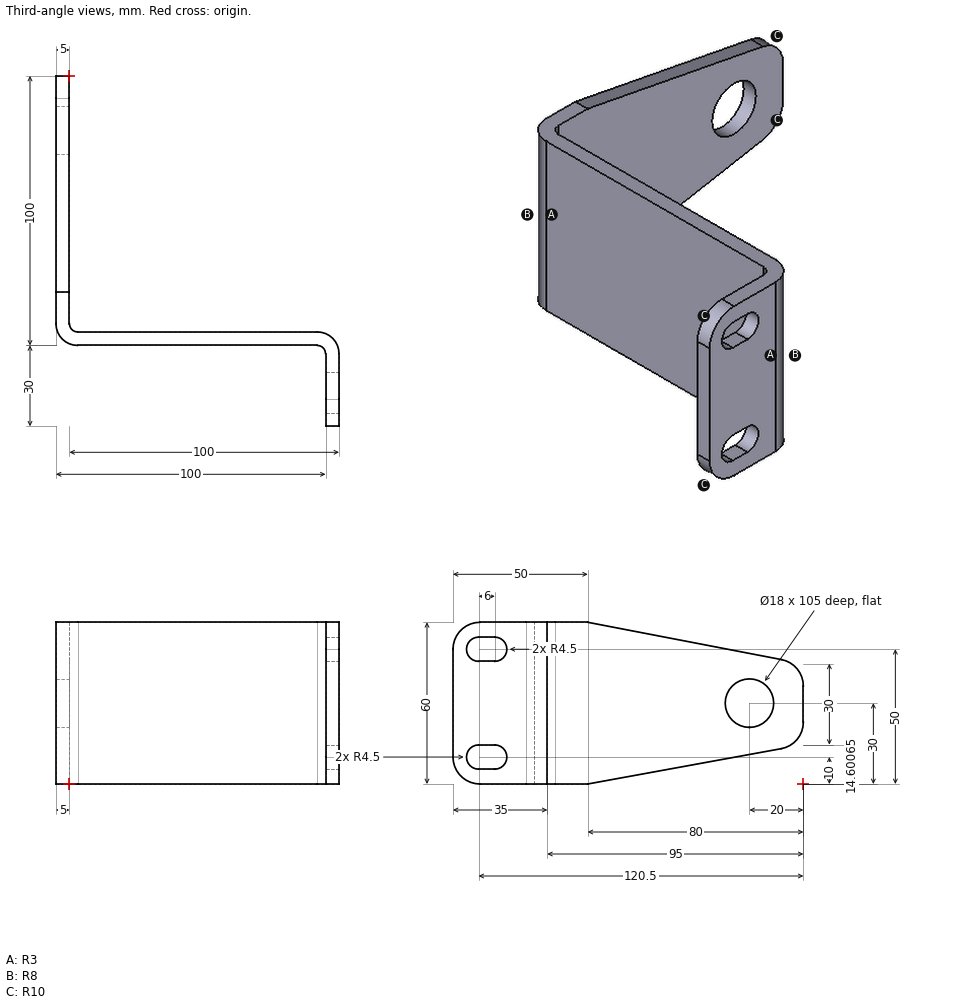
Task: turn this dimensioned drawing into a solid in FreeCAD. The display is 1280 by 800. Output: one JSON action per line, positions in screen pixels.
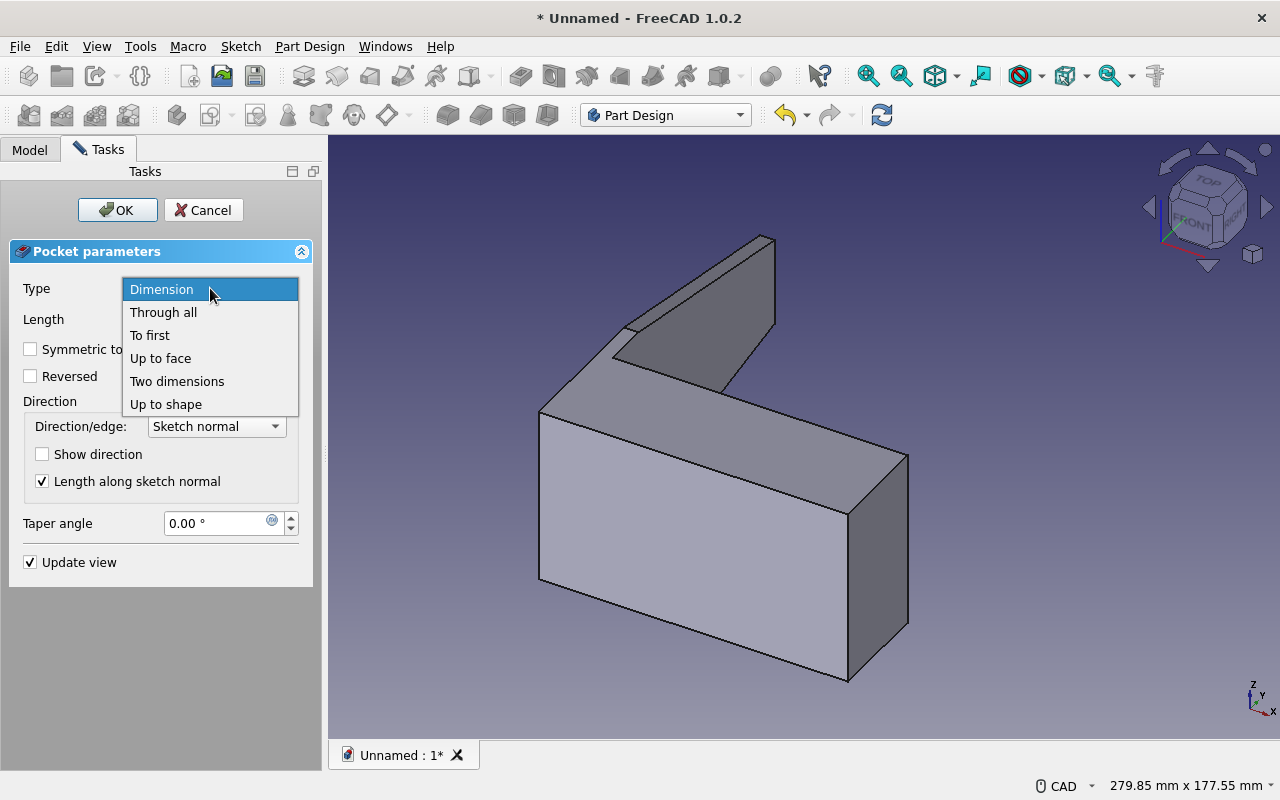
{"action": "left_click", "coordinate": [208, 312]}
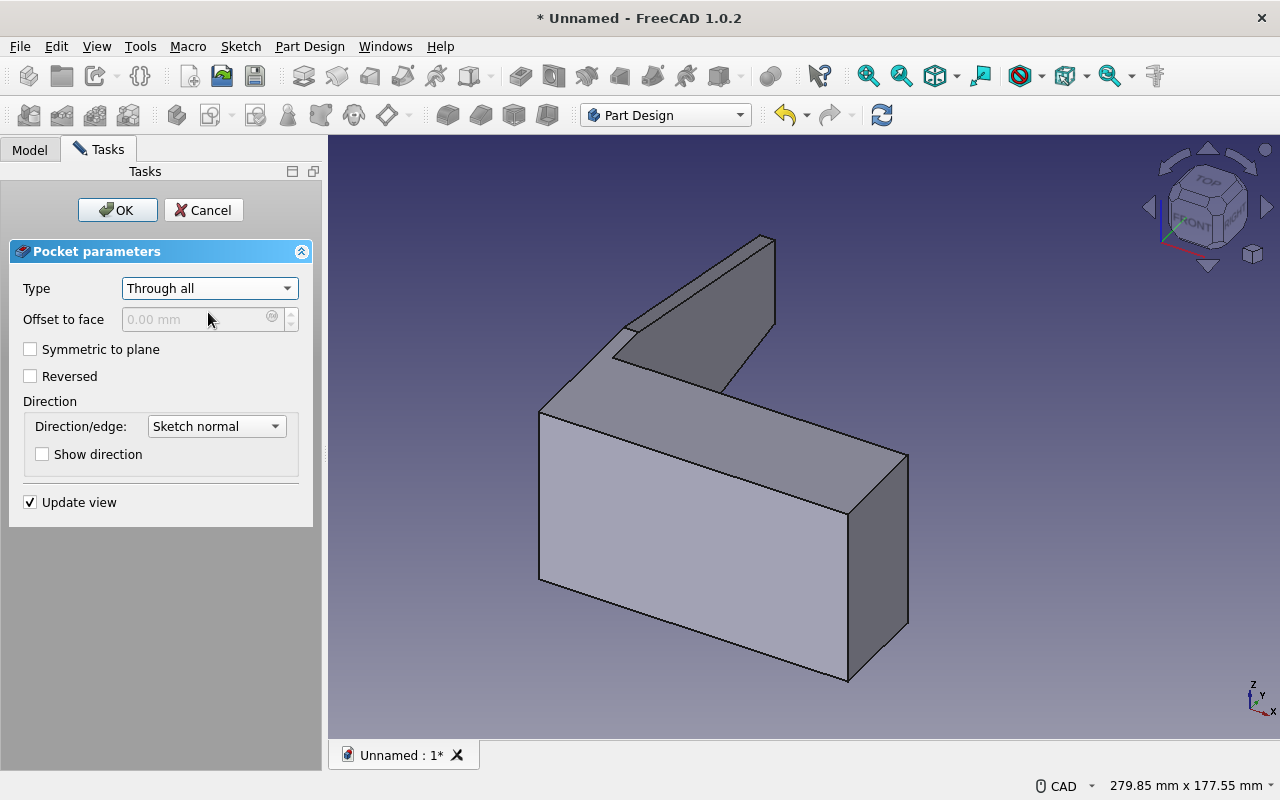
{"action": "left_click", "coordinate": [31, 376]}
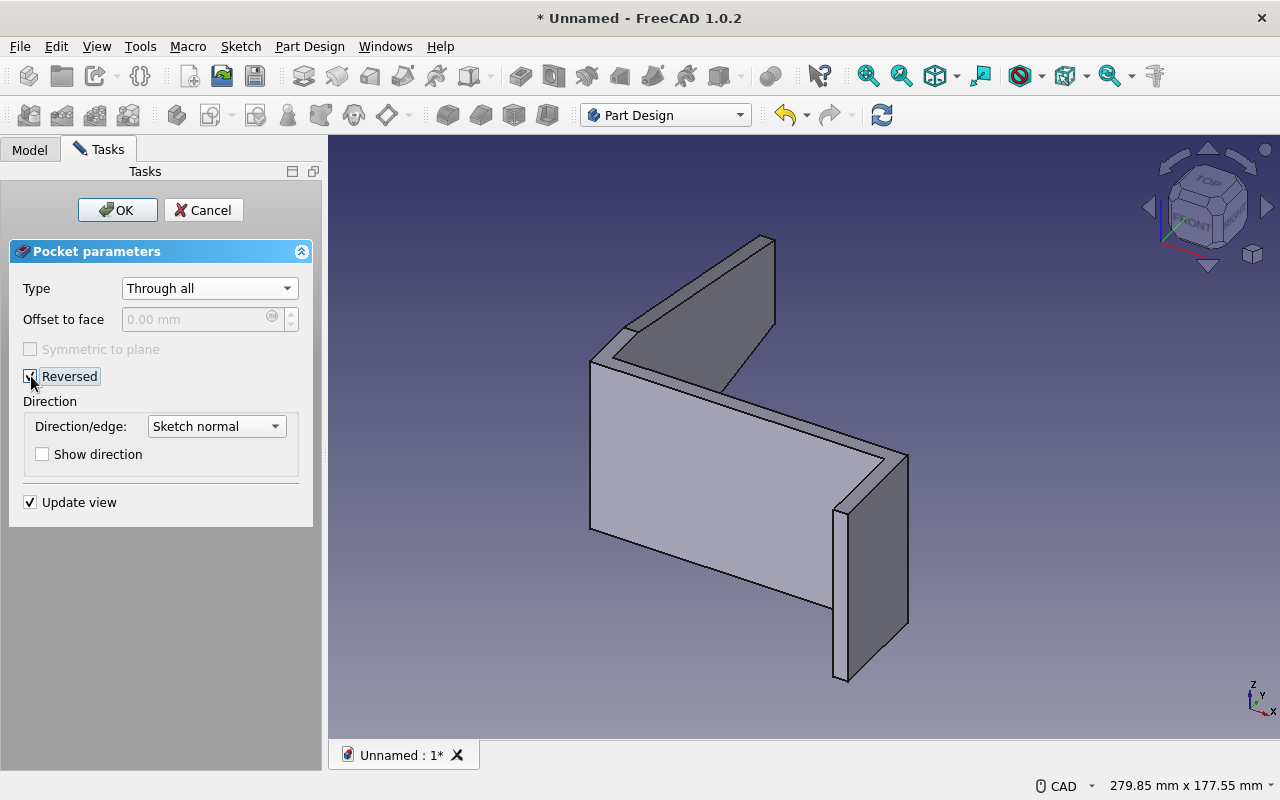
{"action": "left_click", "coordinate": [118, 210]}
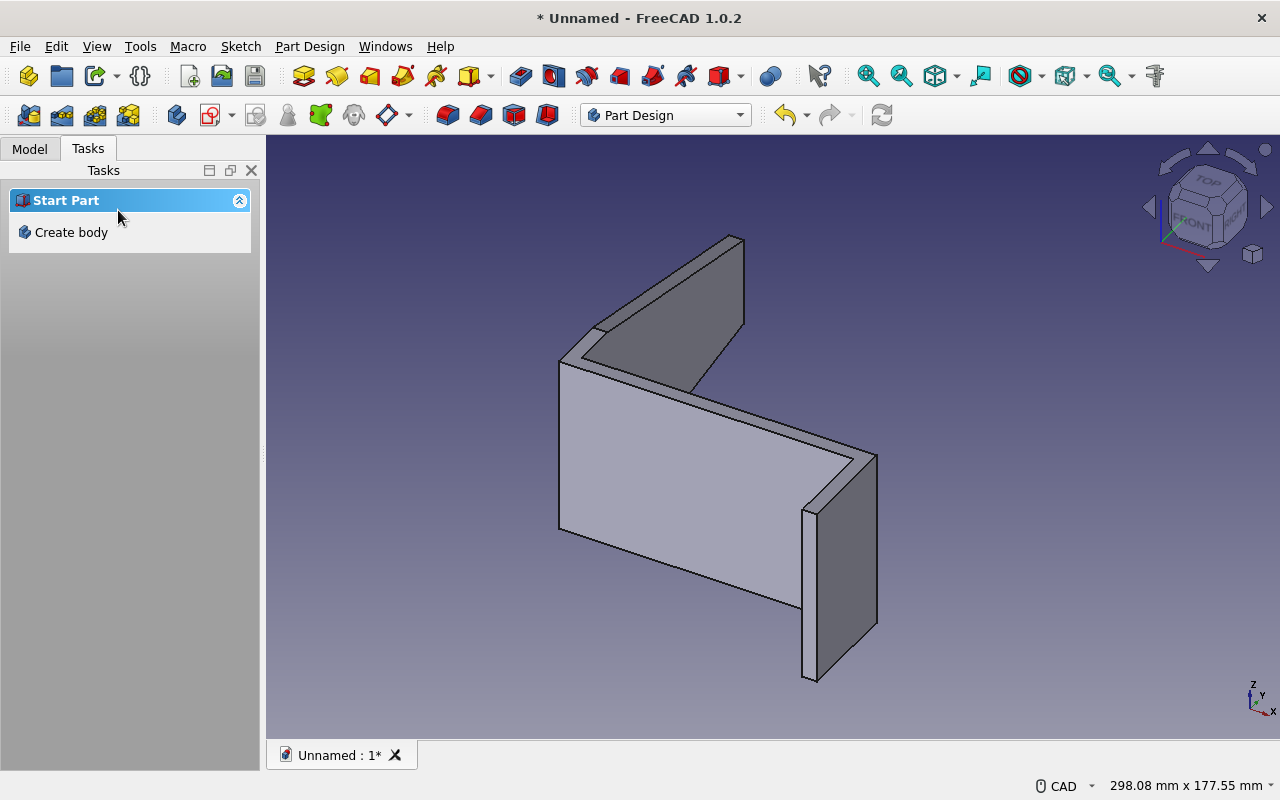
{"action": "key", "text": "6"}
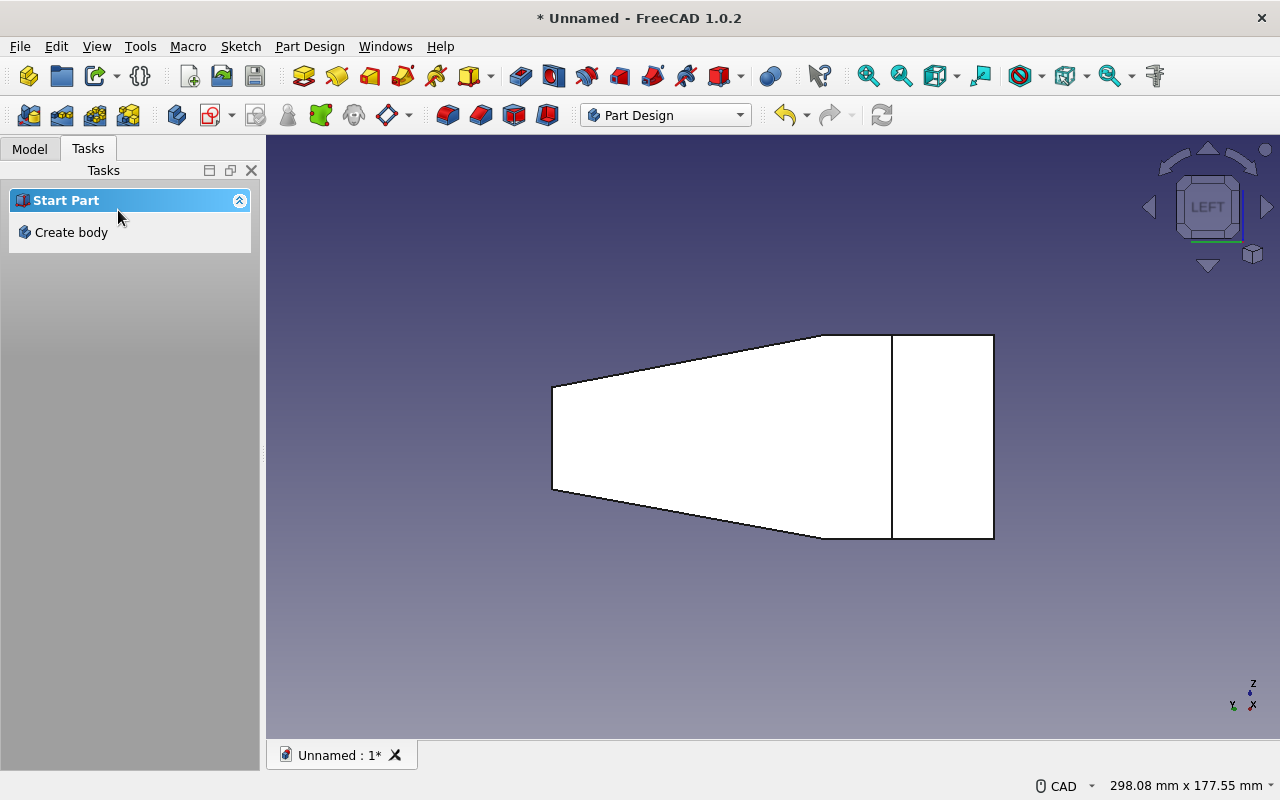
{"action": "left_click", "coordinate": [869, 76]}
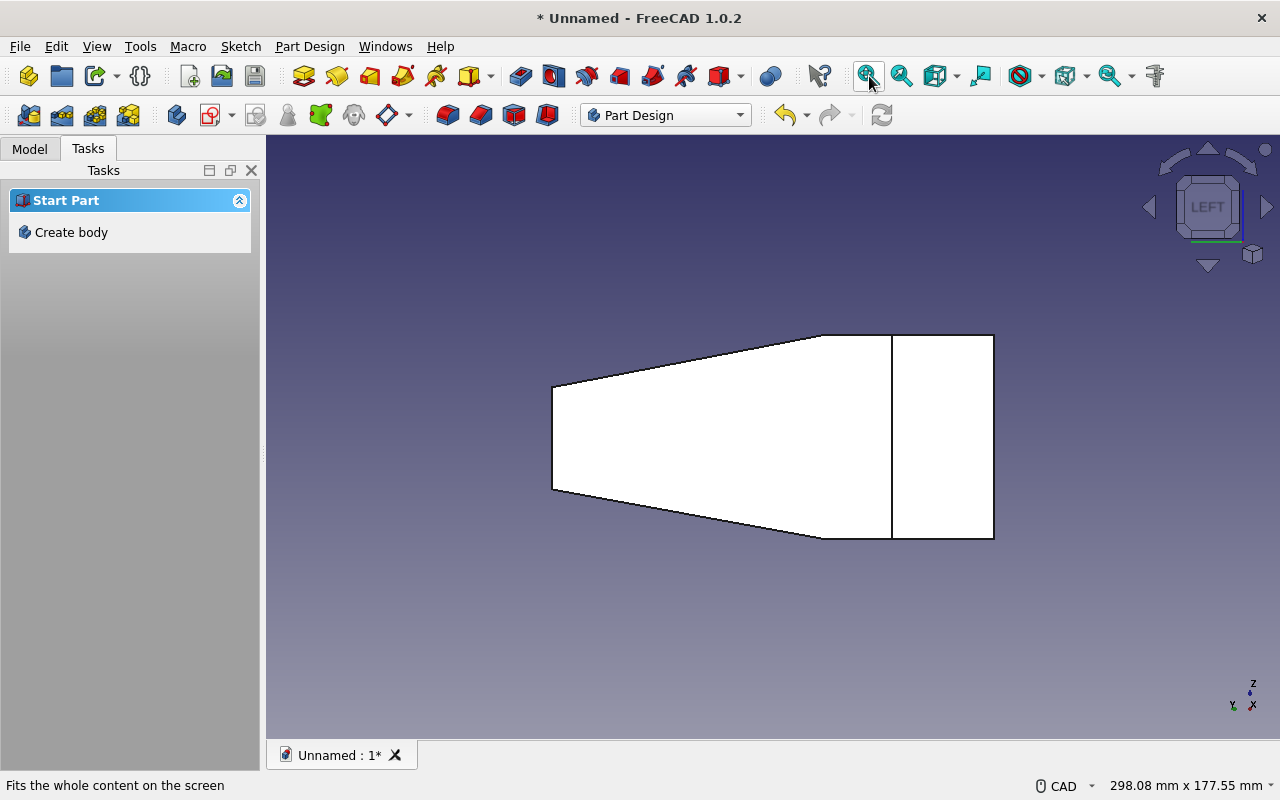
{"action": "left_click", "coordinate": [943, 436]}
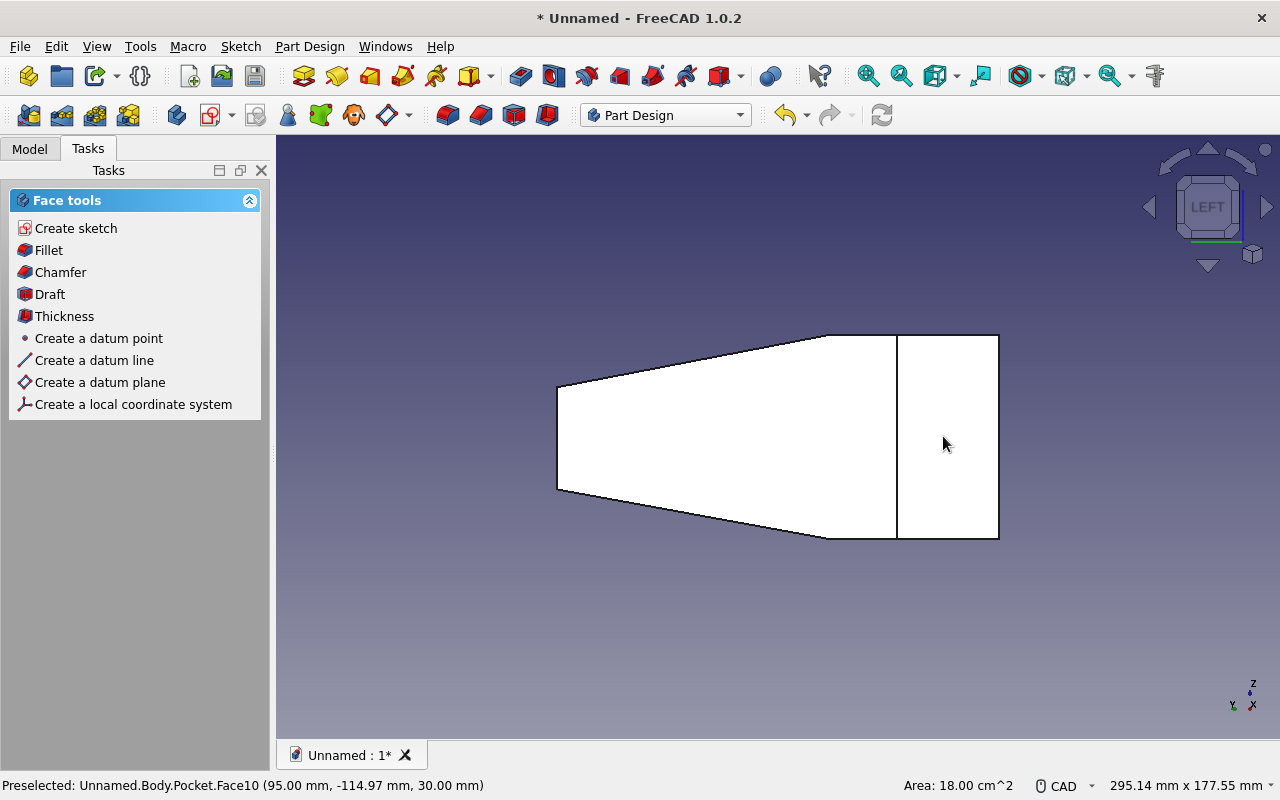
{"action": "left_click", "coordinate": [210, 116]}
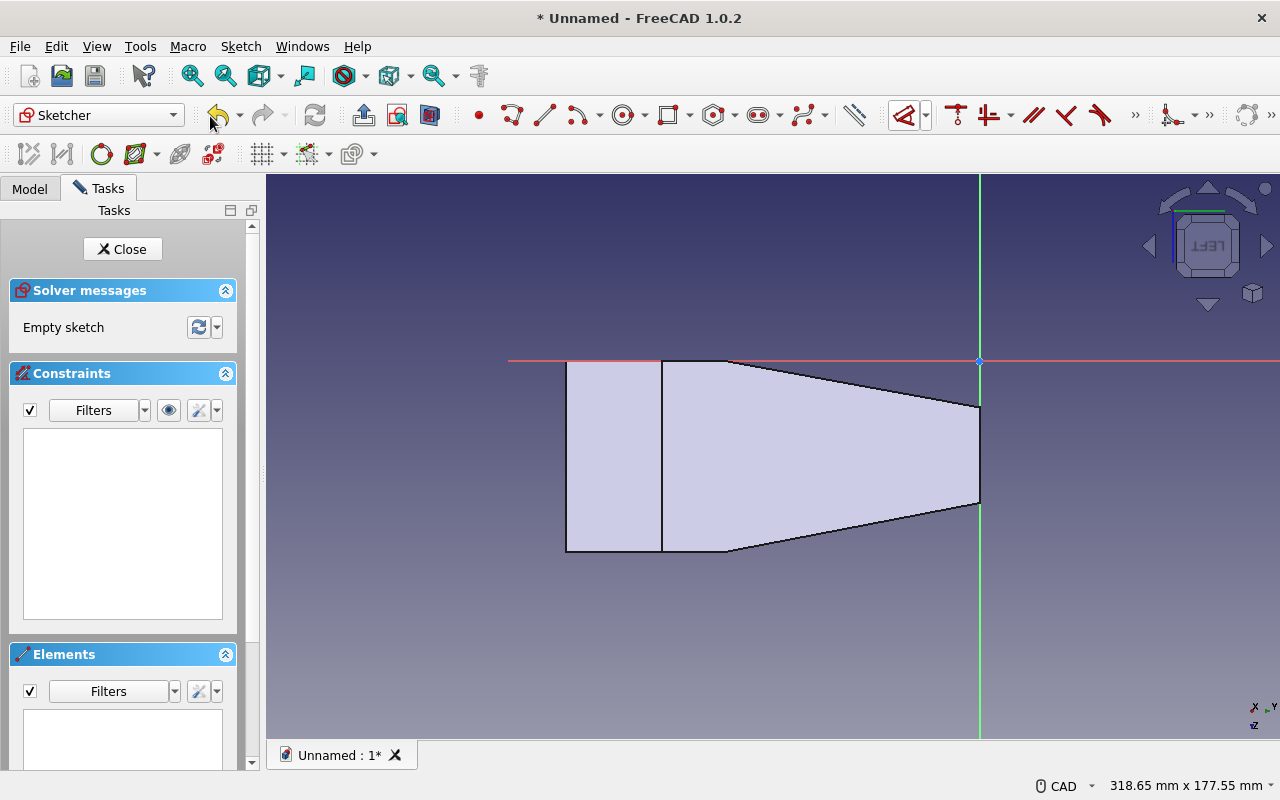
{"action": "scroll", "coordinate": [596, 526], "scroll_direction": "up", "scroll_amount": 12}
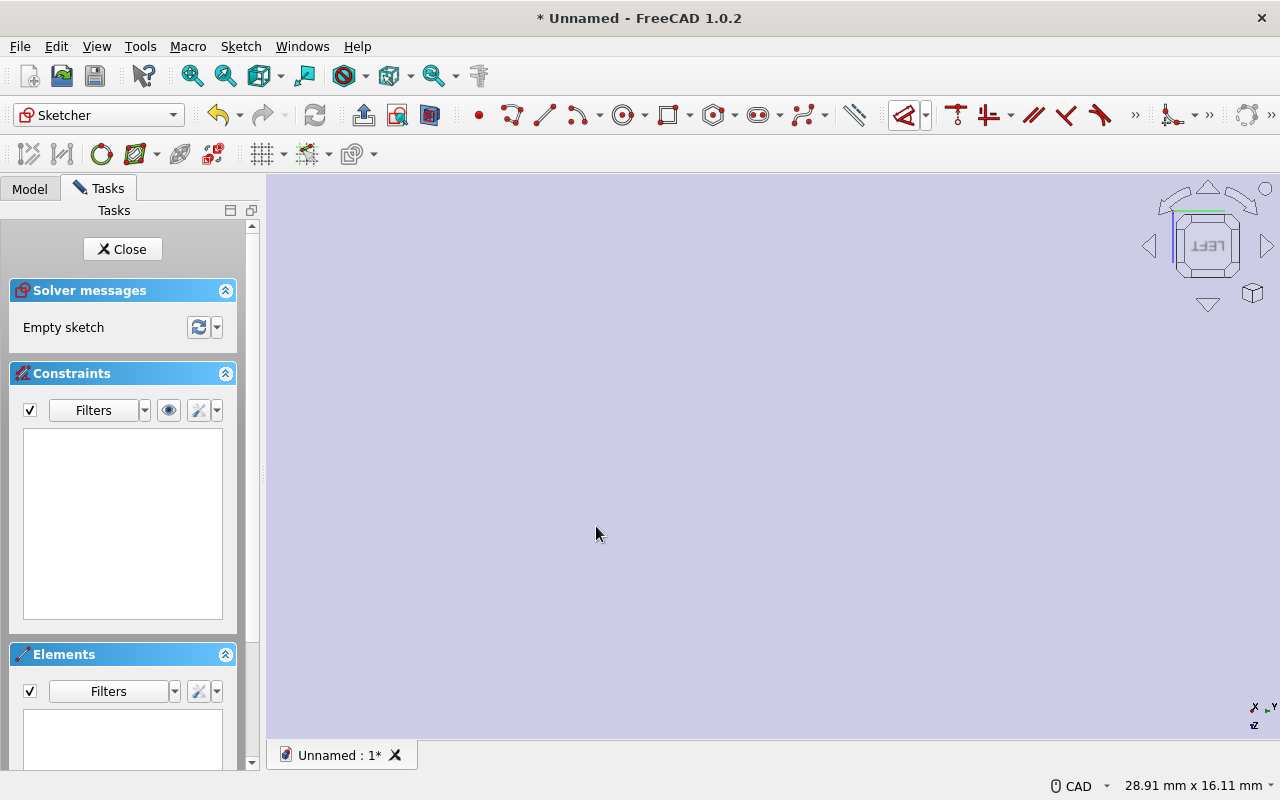
{"action": "left_click", "coordinate": [758, 116]}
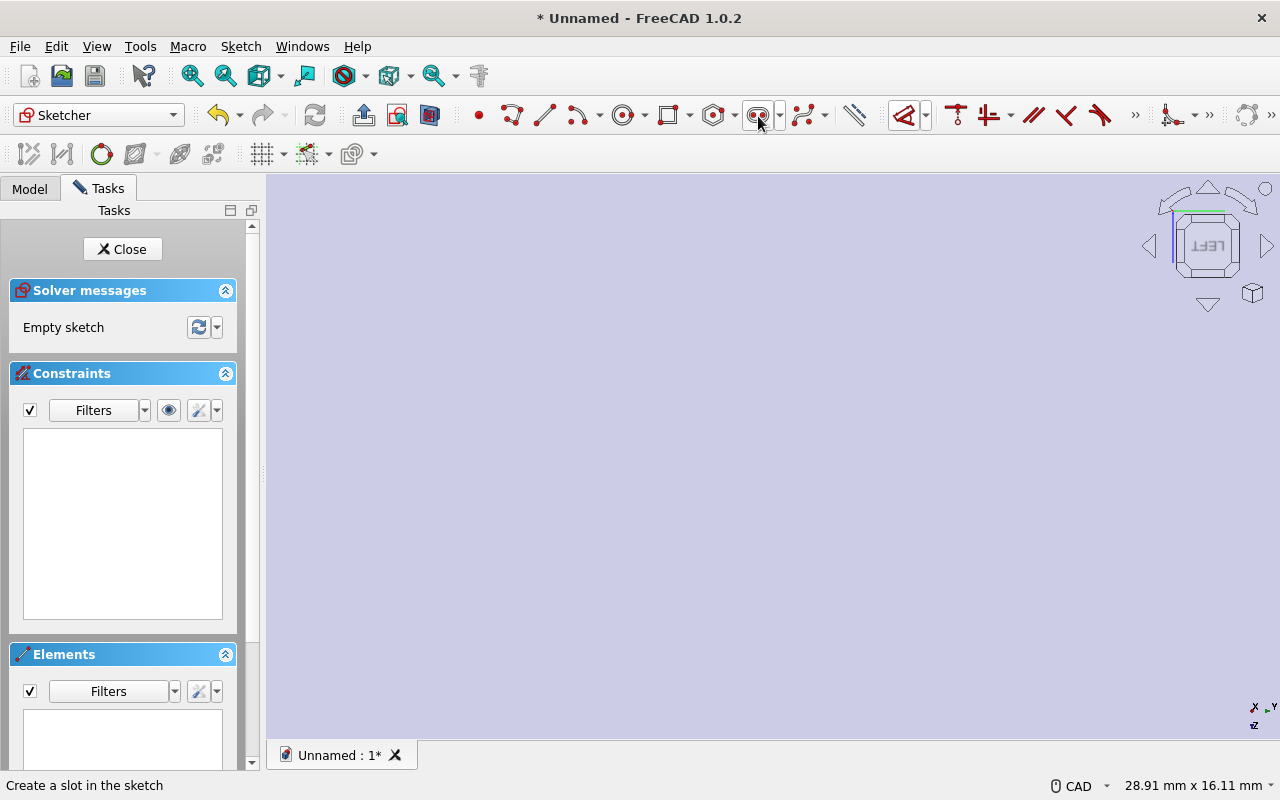
{"action": "left_click", "coordinate": [597, 455]}